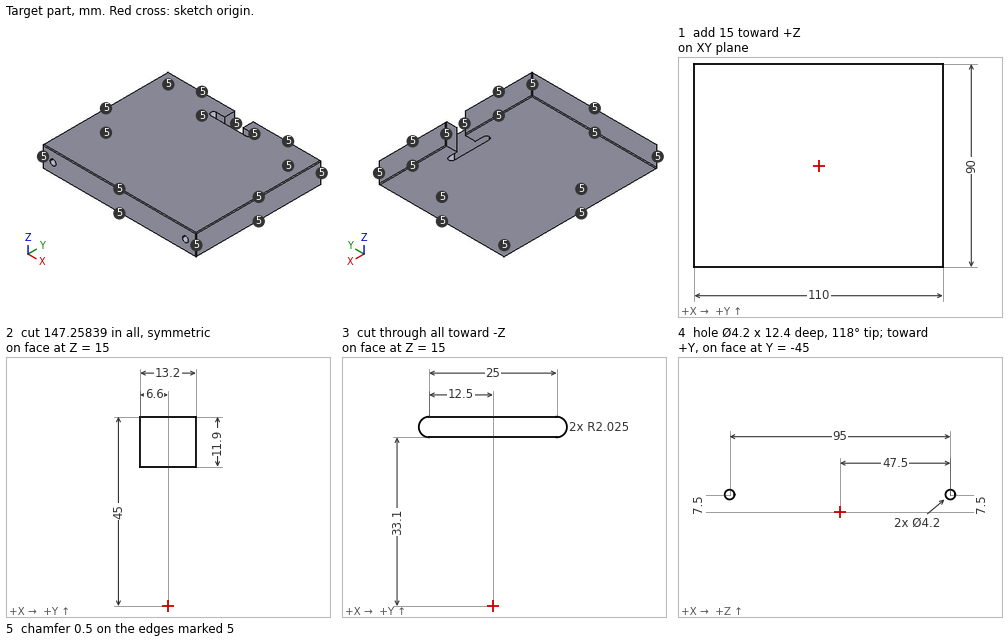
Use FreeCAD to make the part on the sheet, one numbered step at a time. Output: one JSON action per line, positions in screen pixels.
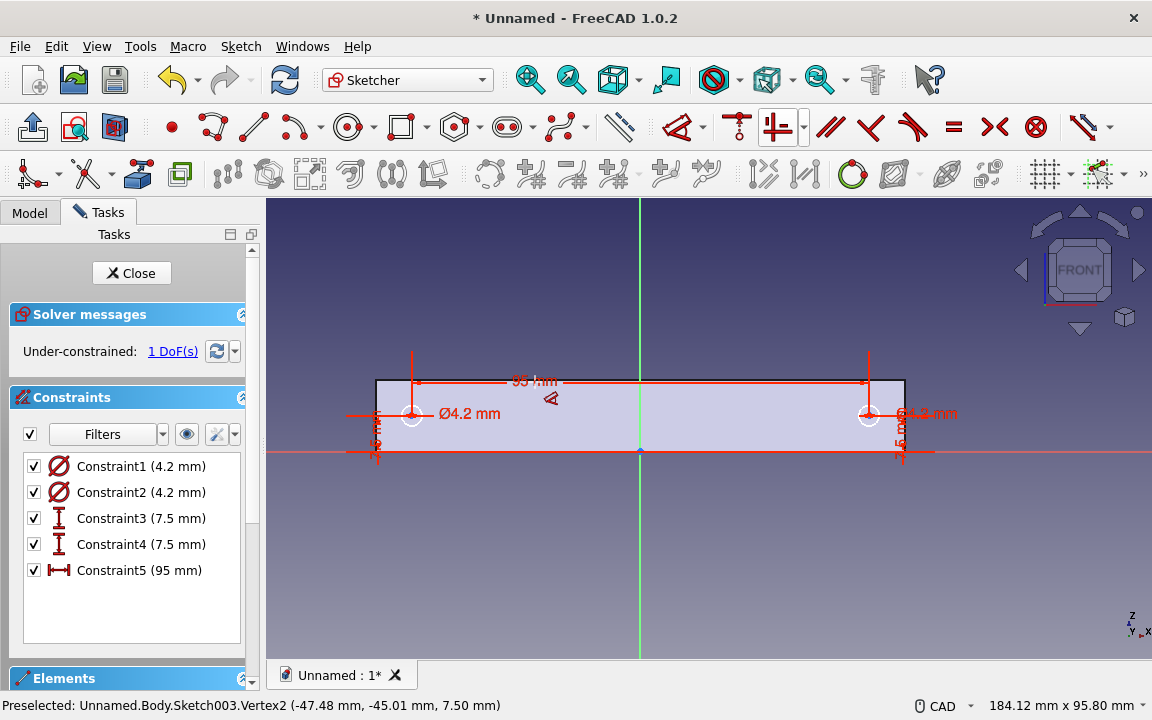
{"action": "left_click", "coordinate": [869, 416]}
{"action": "left_click", "coordinate": [755, 486]}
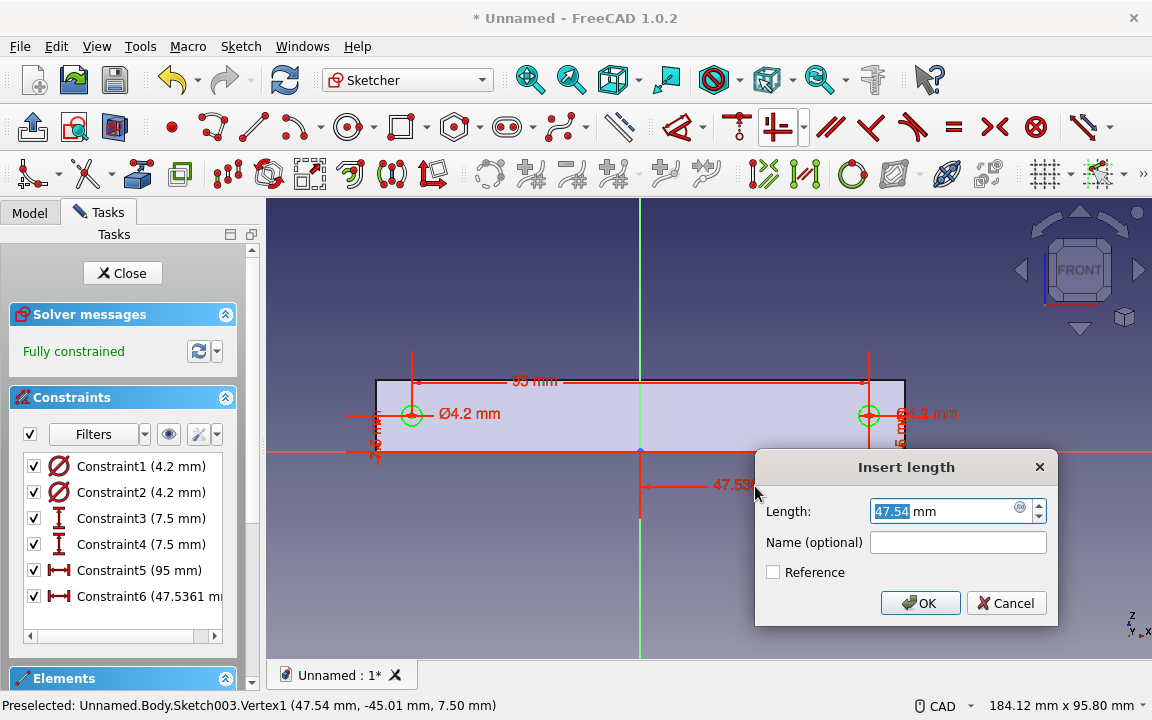
{"action": "type", "text": "47.5"}
{"action": "key", "text": "Return"}
{"action": "key", "text": "Escape"}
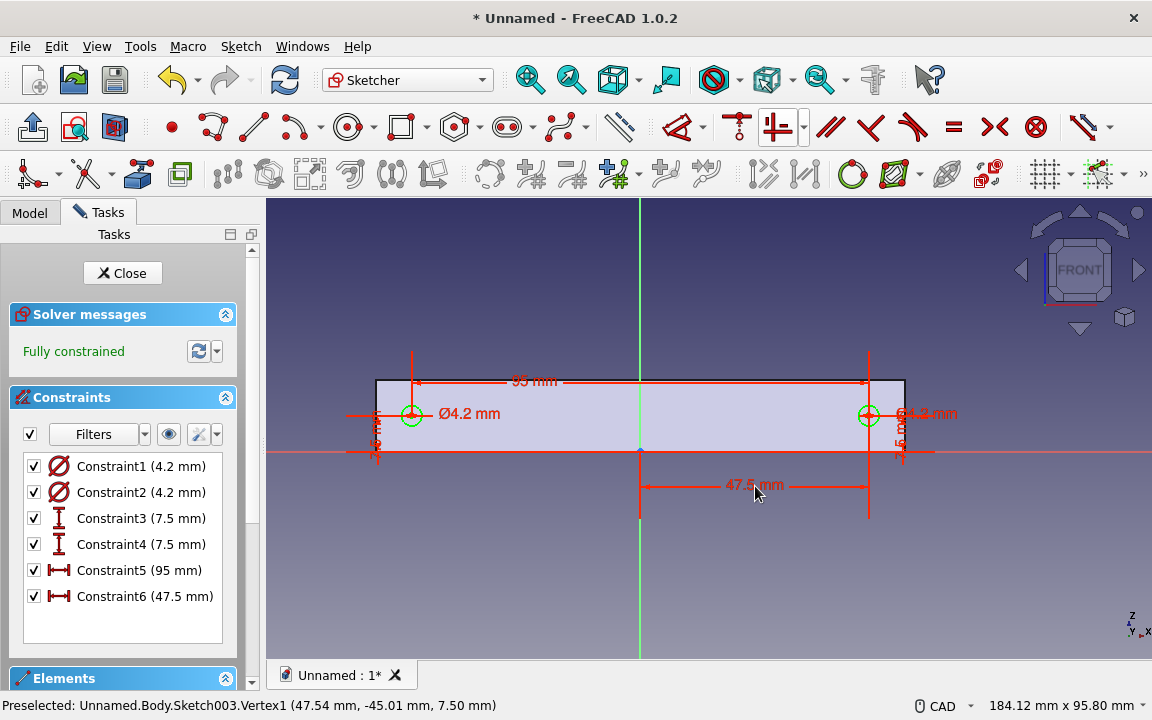
{"action": "left_click", "coordinate": [123, 273]}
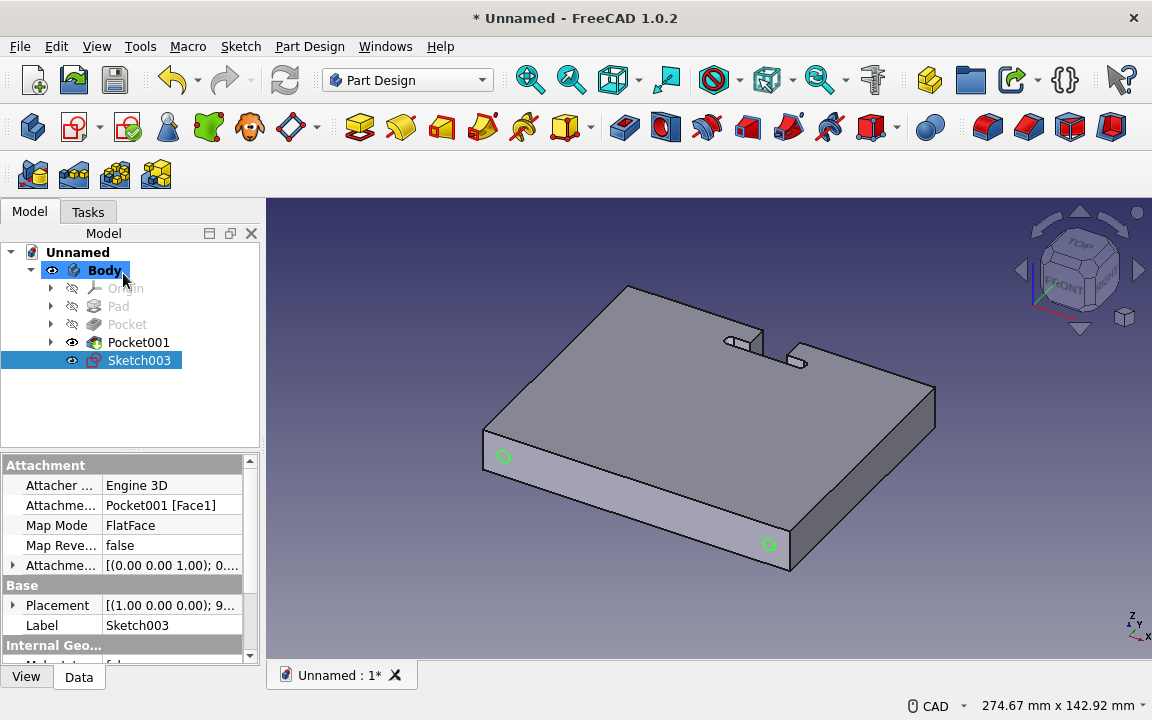
{"action": "left_click", "coordinate": [666, 128]}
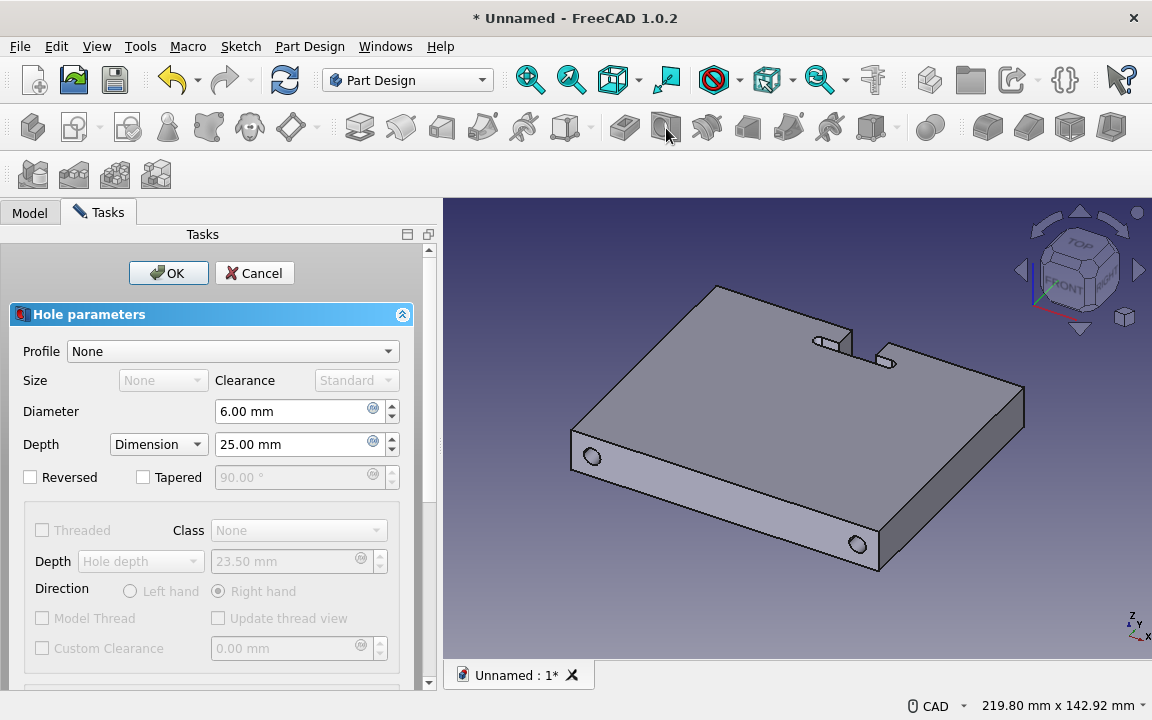
{"action": "triple_click", "coordinate": [300, 412]}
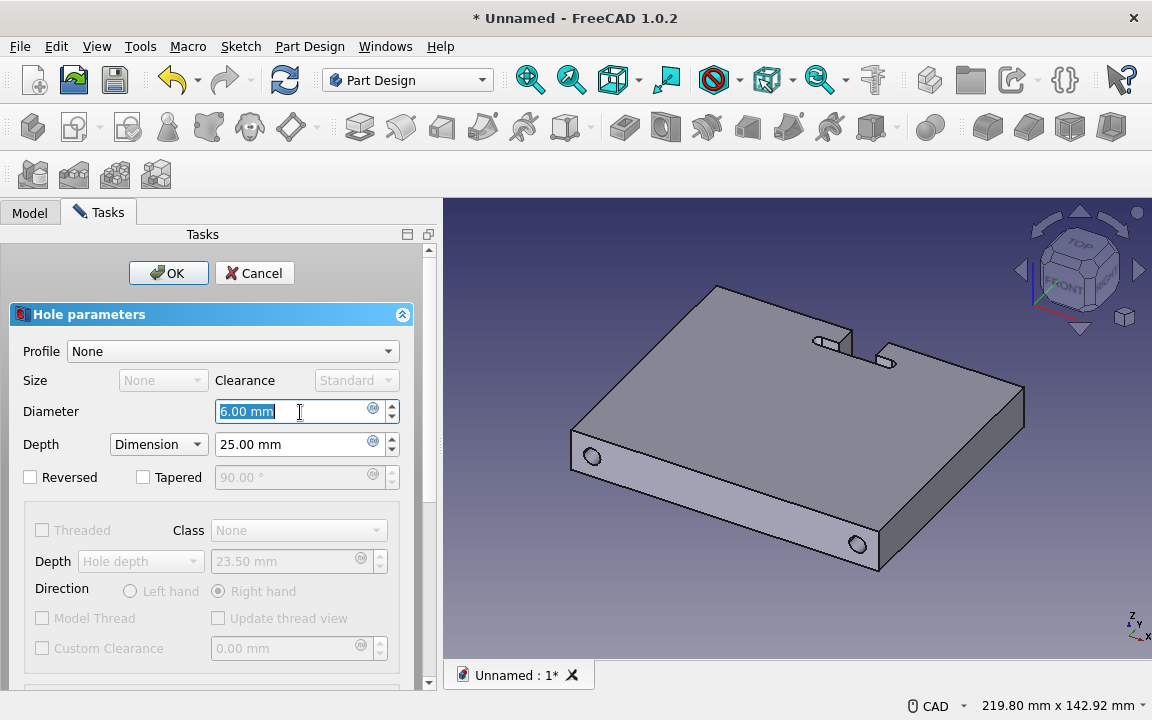
{"action": "type", "text": "4.2"}
{"action": "key", "text": "Tab"}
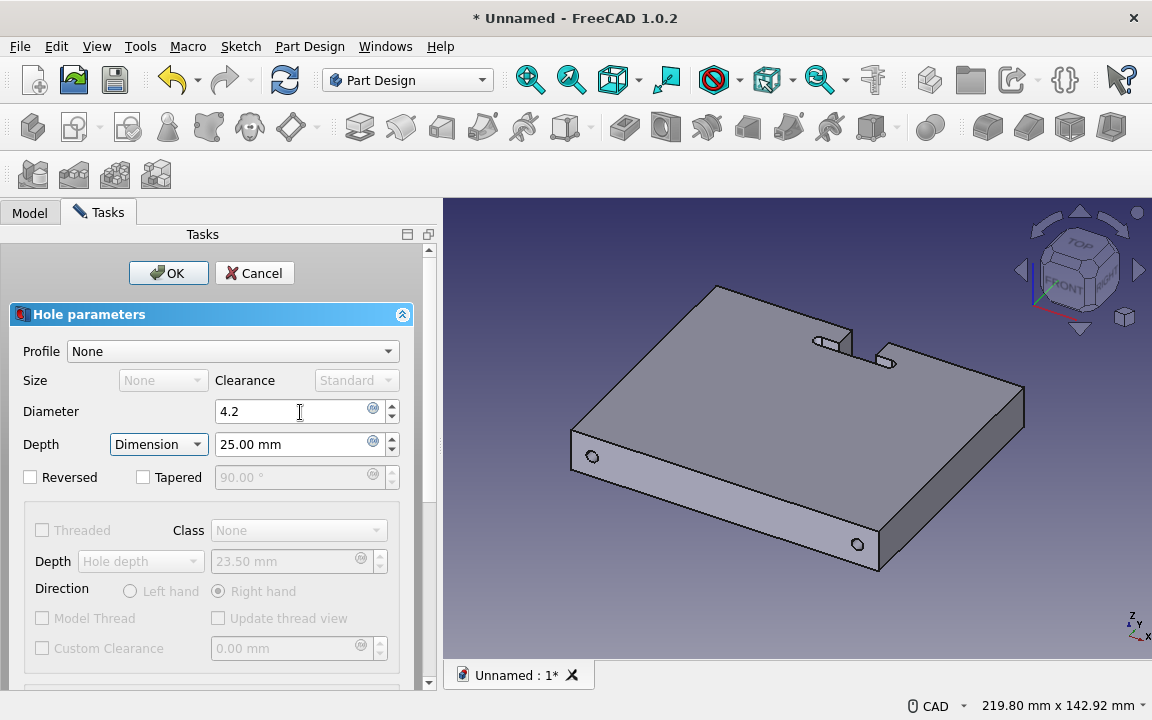
{"action": "triple_click", "coordinate": [300, 444]}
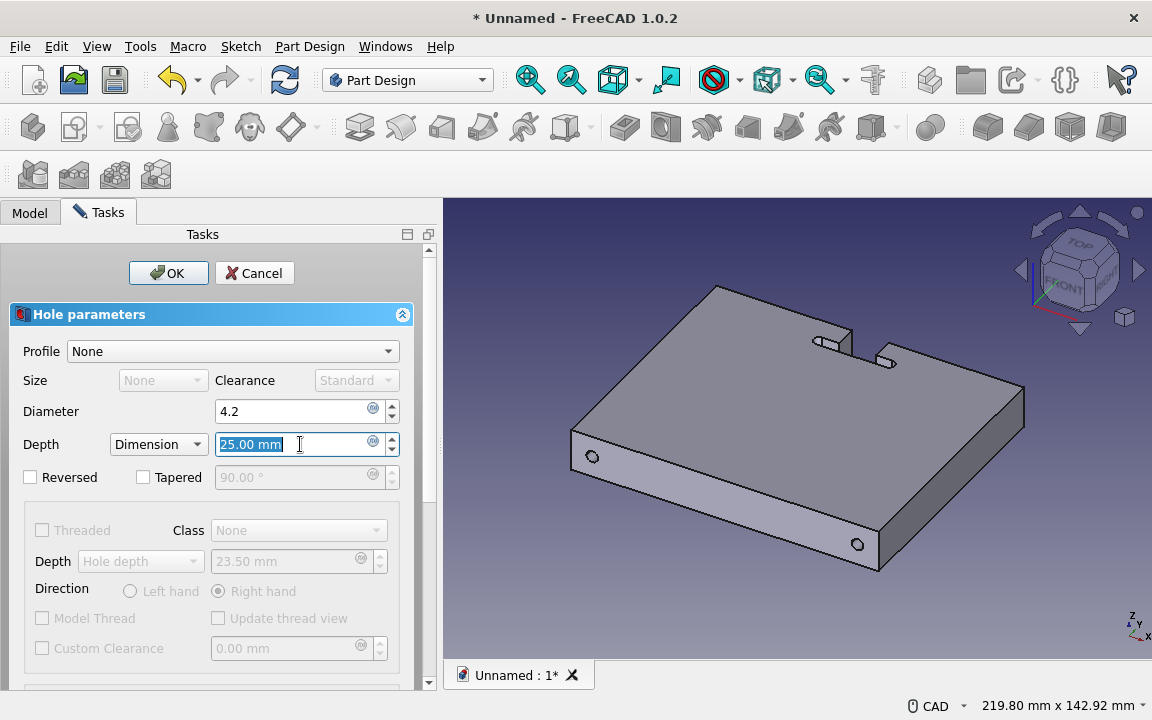
{"action": "type", "text": "12.4"}
{"action": "key", "text": "Tab"}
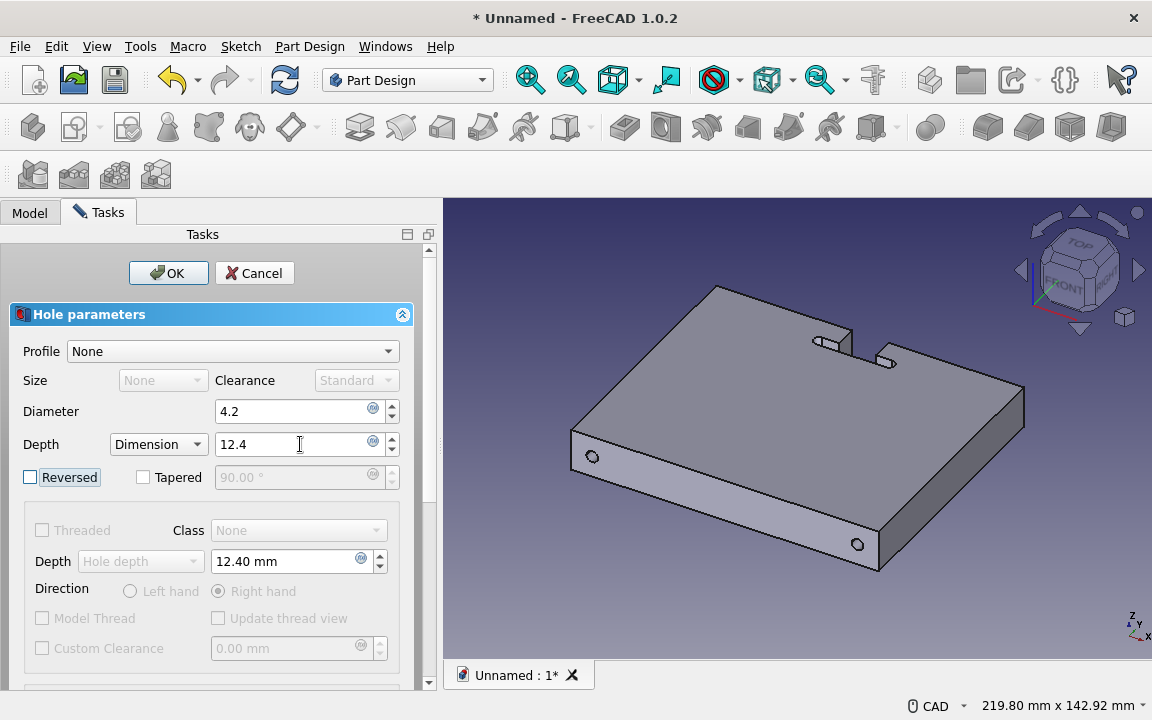
{"action": "left_click", "coordinate": [169, 273]}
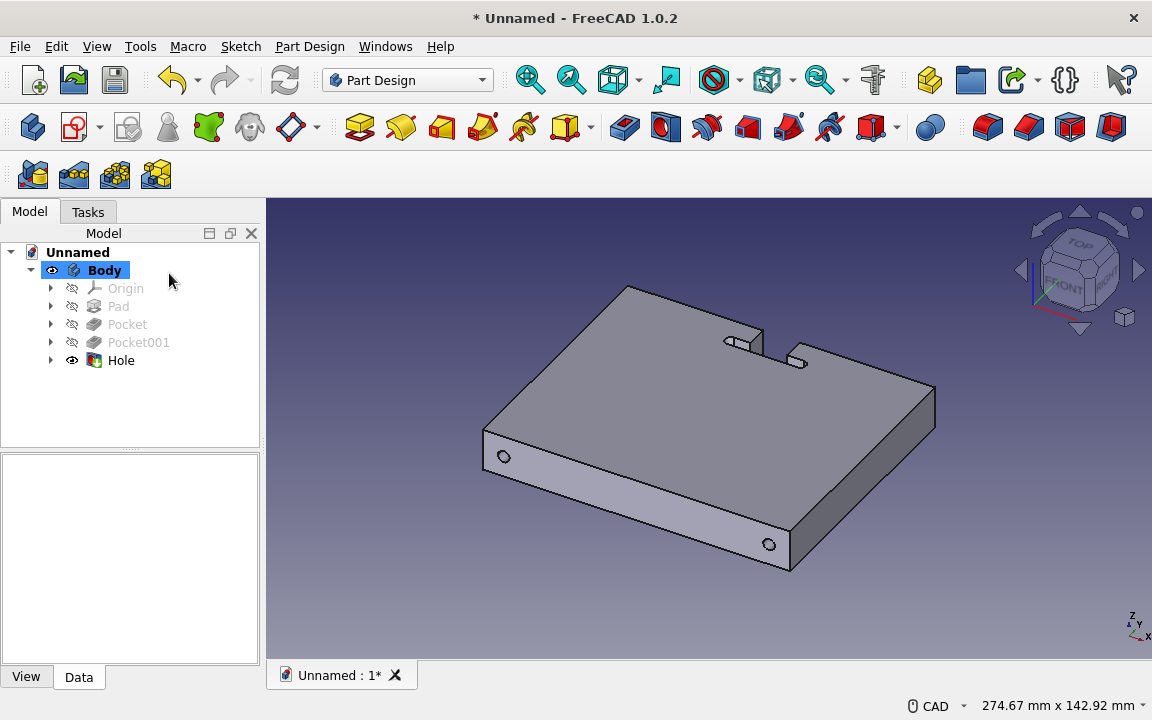
{"action": "left_click", "coordinate": [904, 437]}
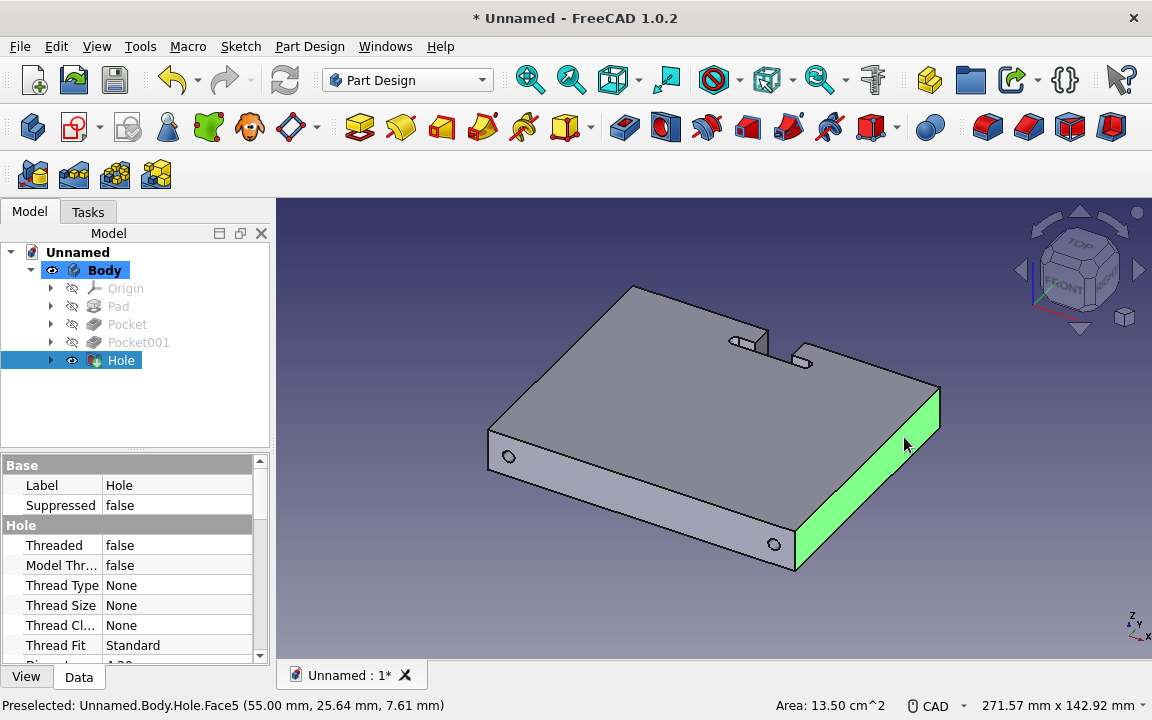
{"action": "left_click", "coordinate": [641, 480], "text": "ctrl"}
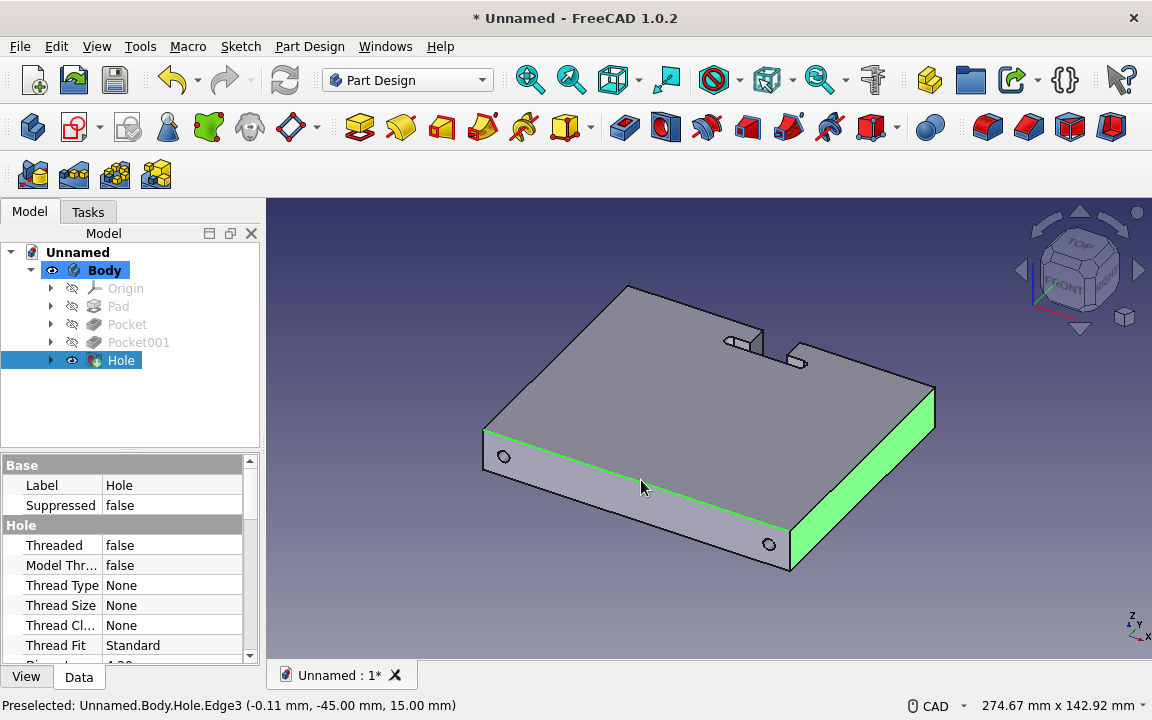
{"action": "key", "text": "0"}